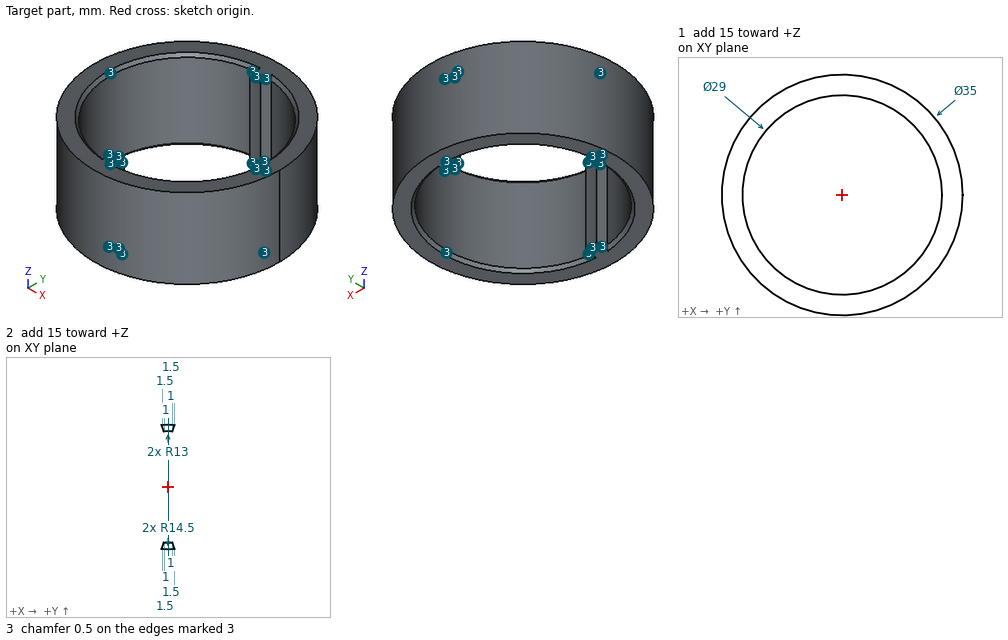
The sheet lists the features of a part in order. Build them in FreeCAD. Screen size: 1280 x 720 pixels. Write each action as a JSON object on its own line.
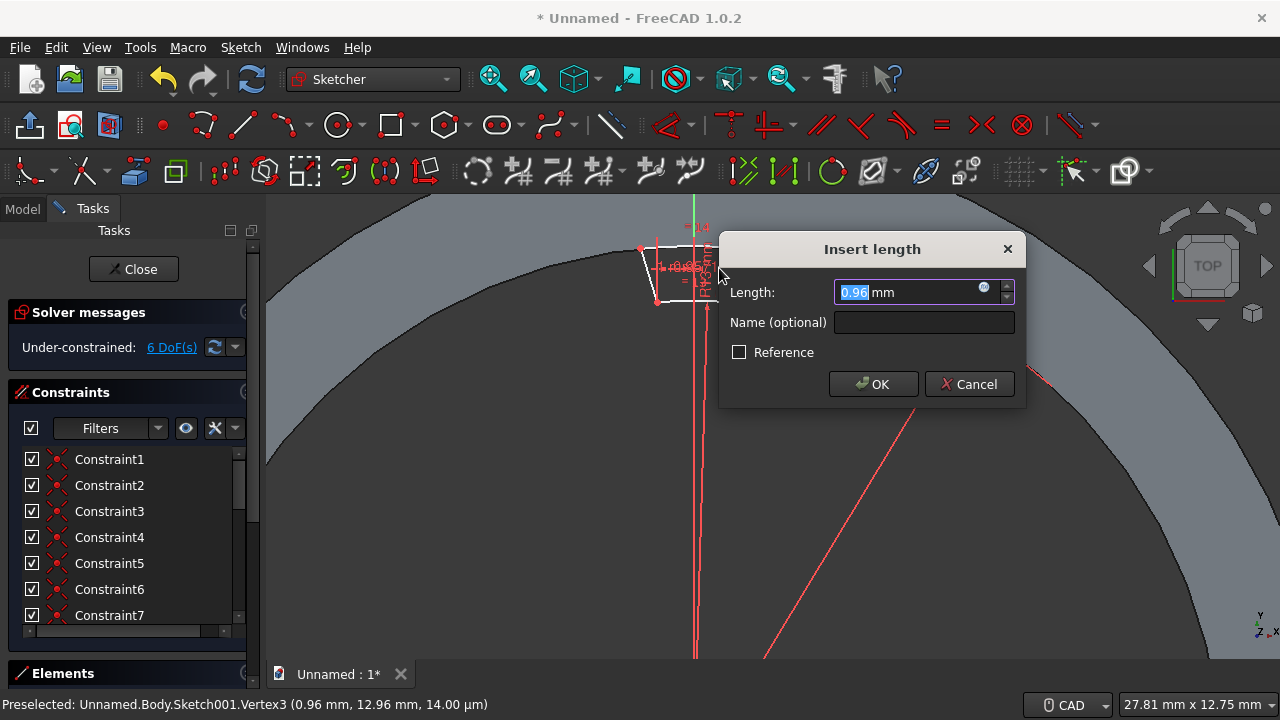
{"action": "type", "text": "1"}
{"action": "key", "text": "Return"}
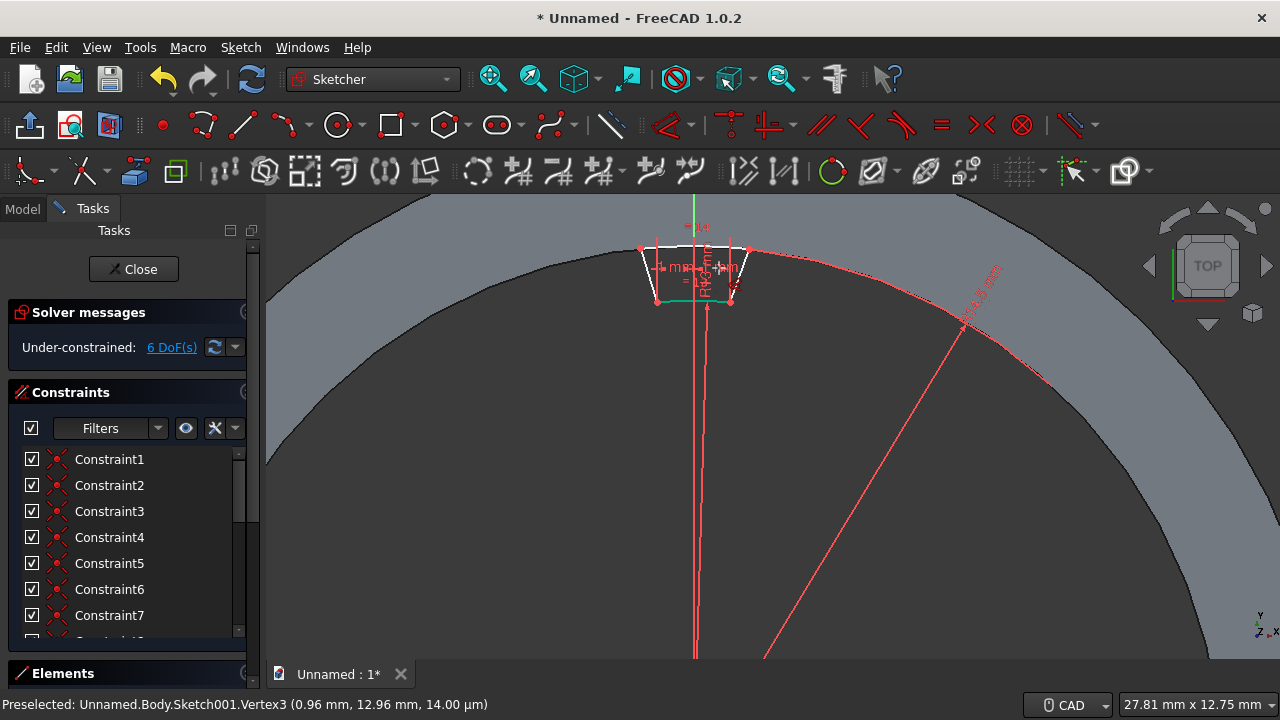
{"action": "scroll", "coordinate": [709, 276], "scroll_direction": "down", "scroll_amount": 6}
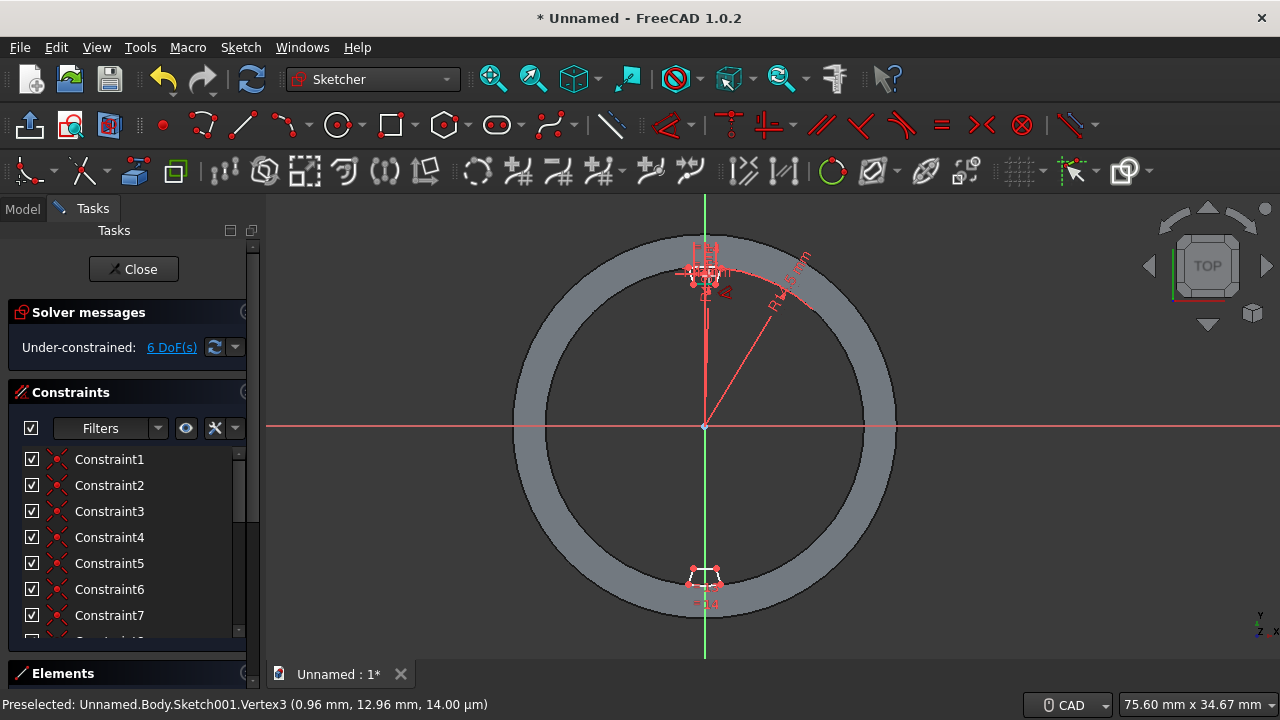
{"action": "scroll", "coordinate": [716, 569], "scroll_direction": "up", "scroll_amount": 7}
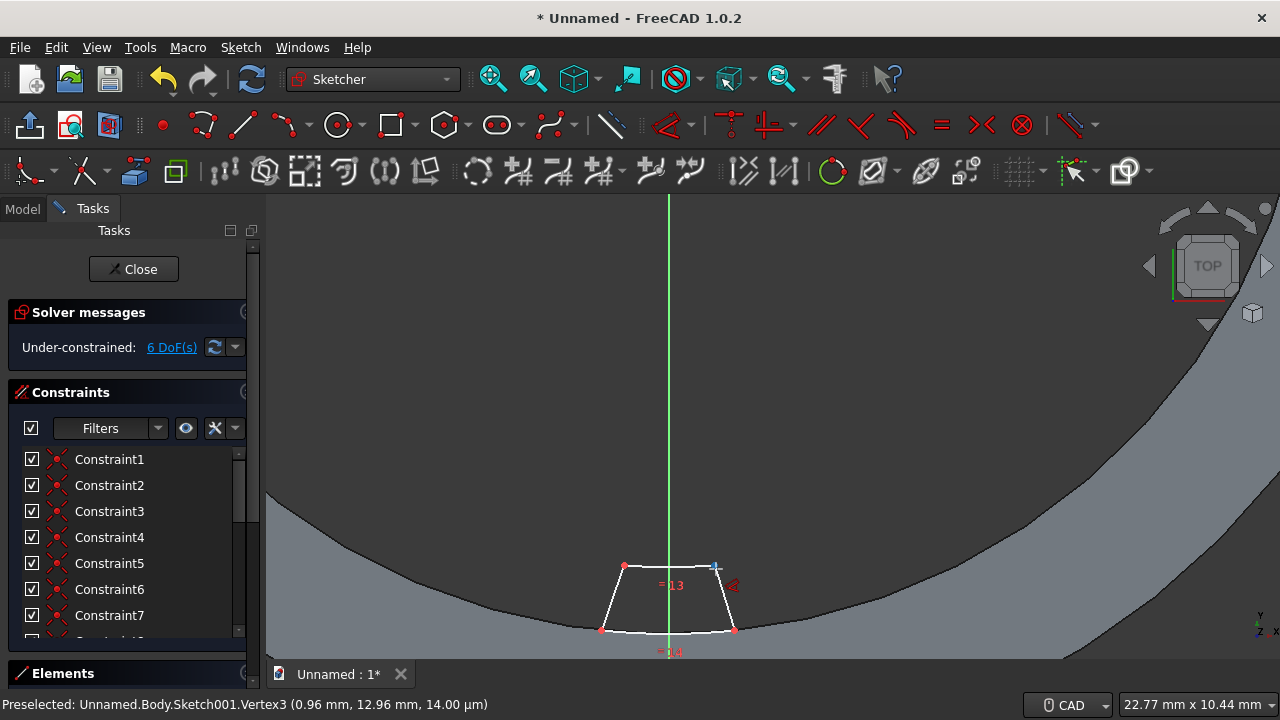
{"action": "left_click", "coordinate": [715, 565]}
{"action": "left_click", "coordinate": [692, 599]}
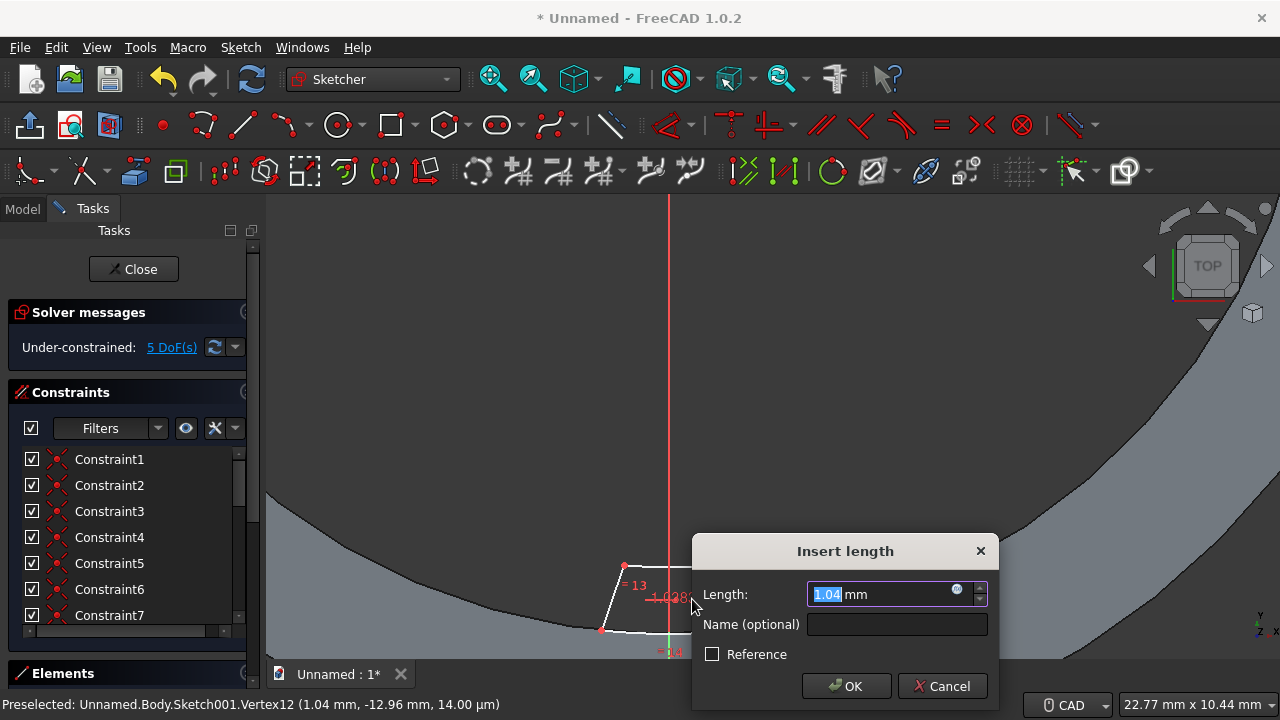
{"action": "type", "text": "1"}
{"action": "key", "text": "Return"}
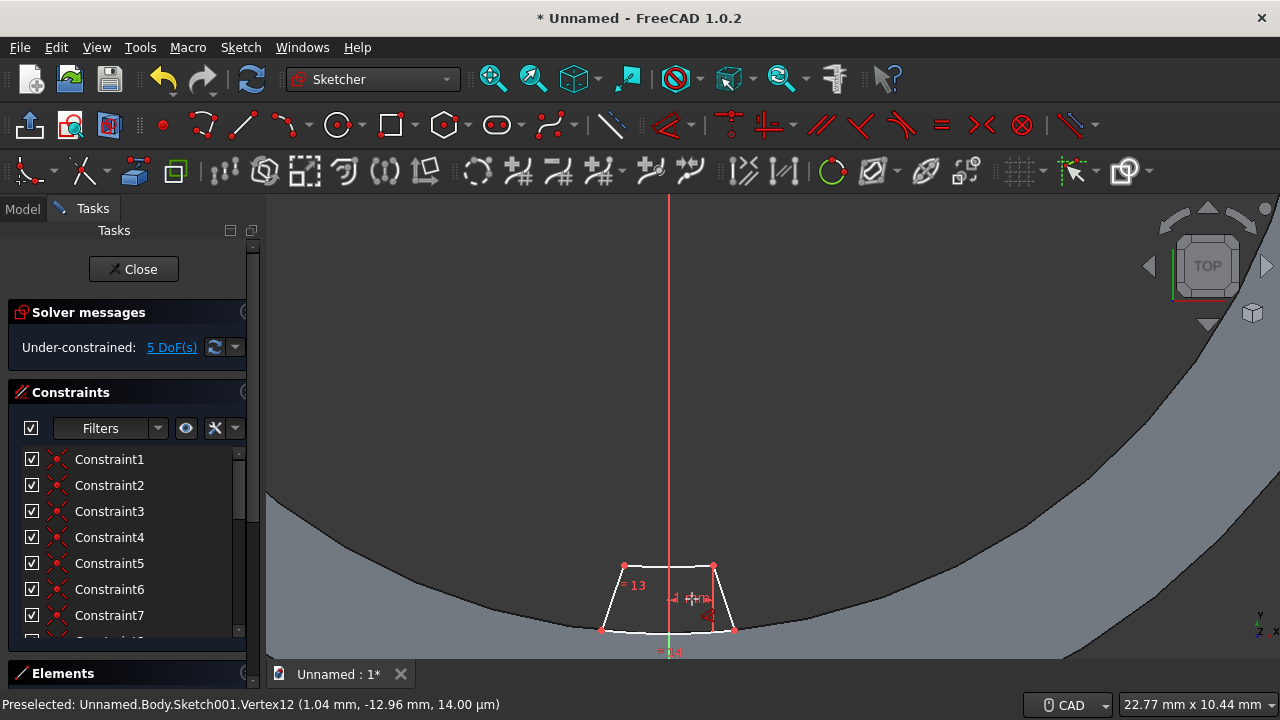
{"action": "left_click", "coordinate": [624, 565]}
{"action": "left_click", "coordinate": [646, 599]}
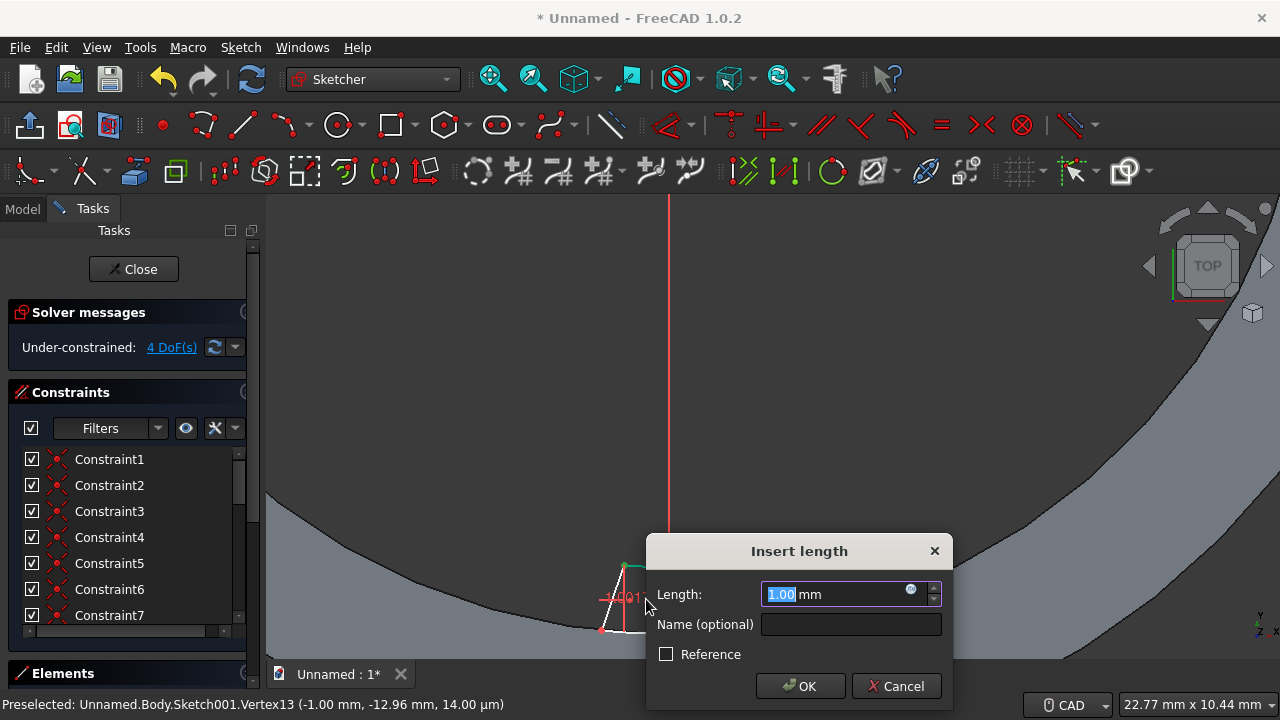
{"action": "type", "text": "1"}
{"action": "key", "text": "Return"}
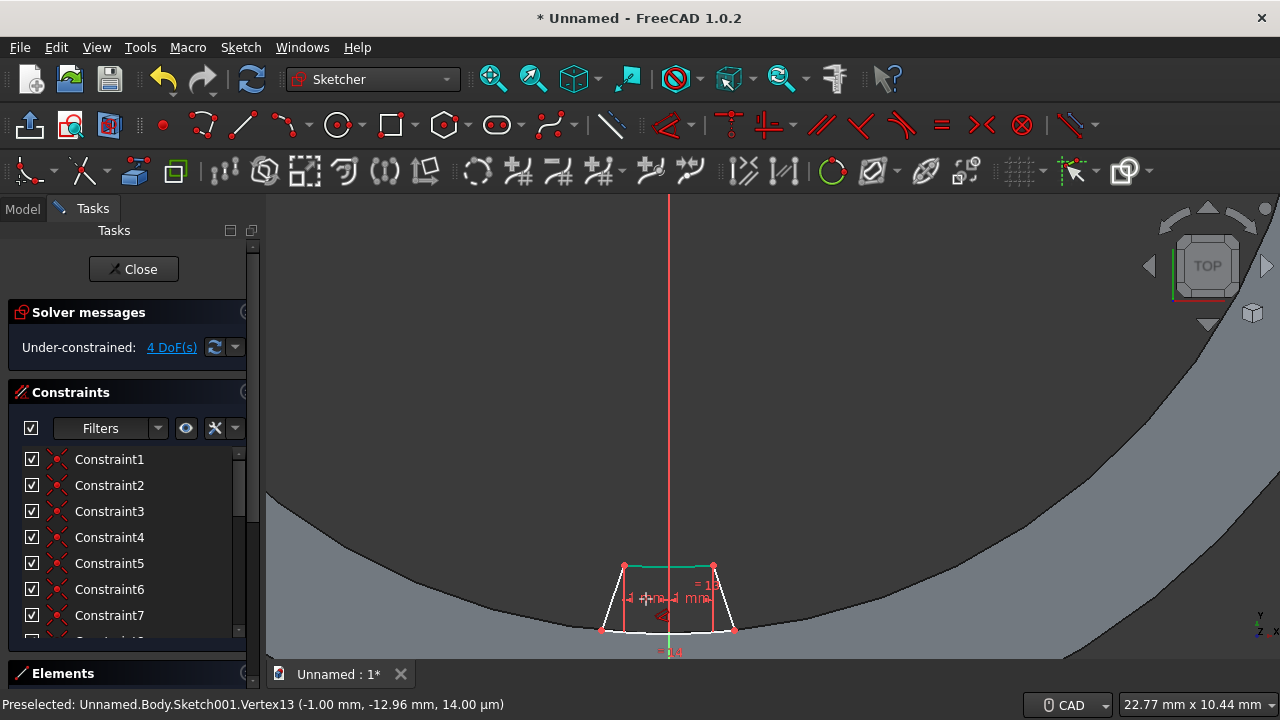
{"action": "scroll", "coordinate": [716, 570], "scroll_direction": "down", "scroll_amount": 7}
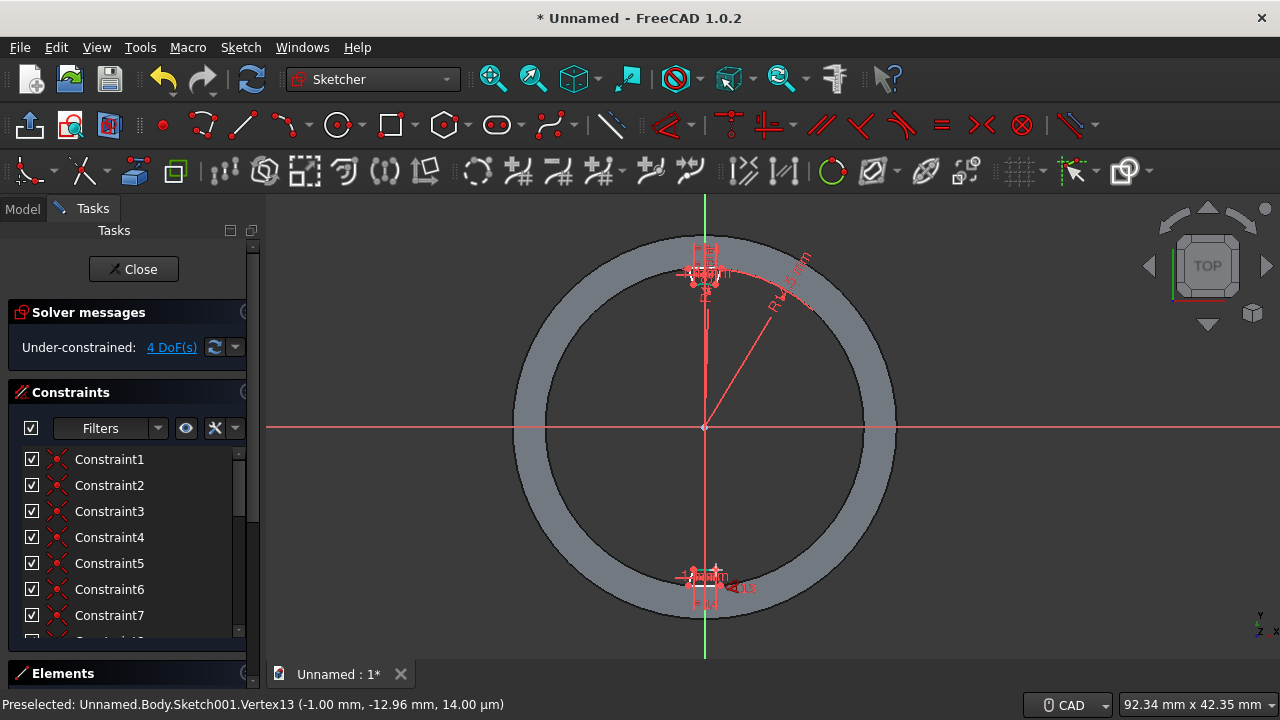
{"action": "scroll", "coordinate": [689, 269], "scroll_direction": "up", "scroll_amount": 5}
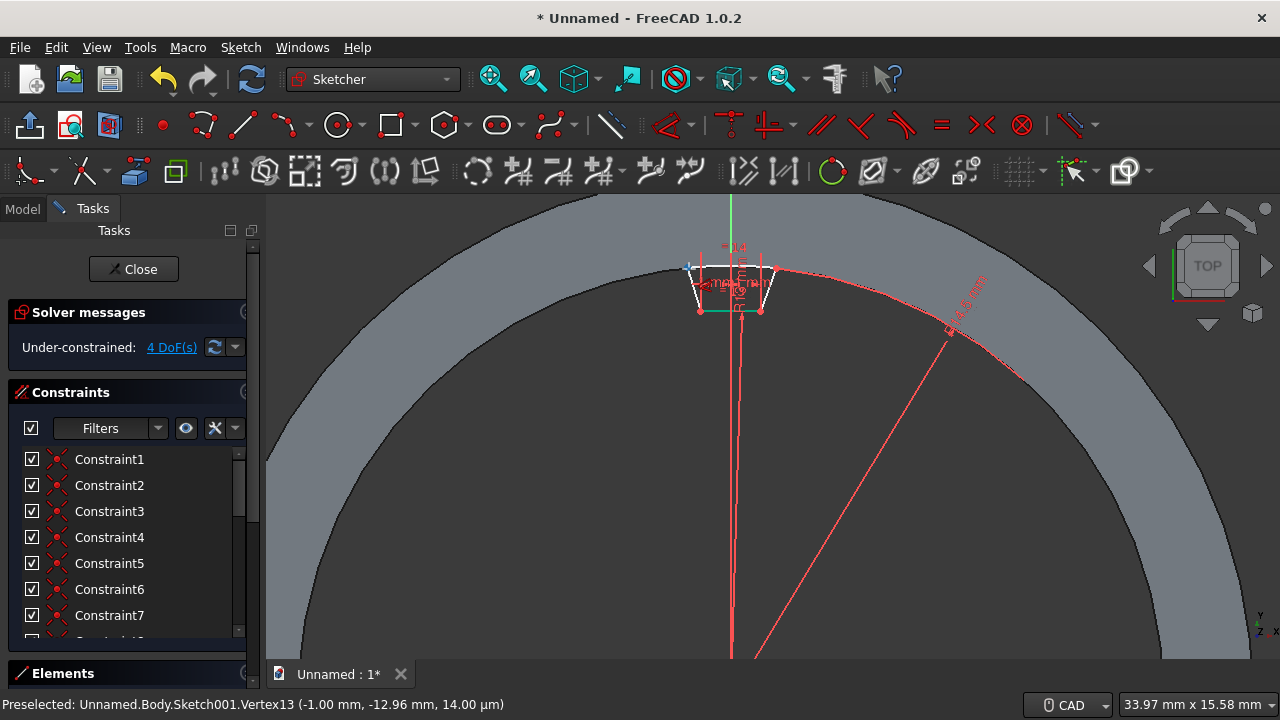
{"action": "left_click", "coordinate": [688, 268]}
{"action": "left_click", "coordinate": [709, 234]}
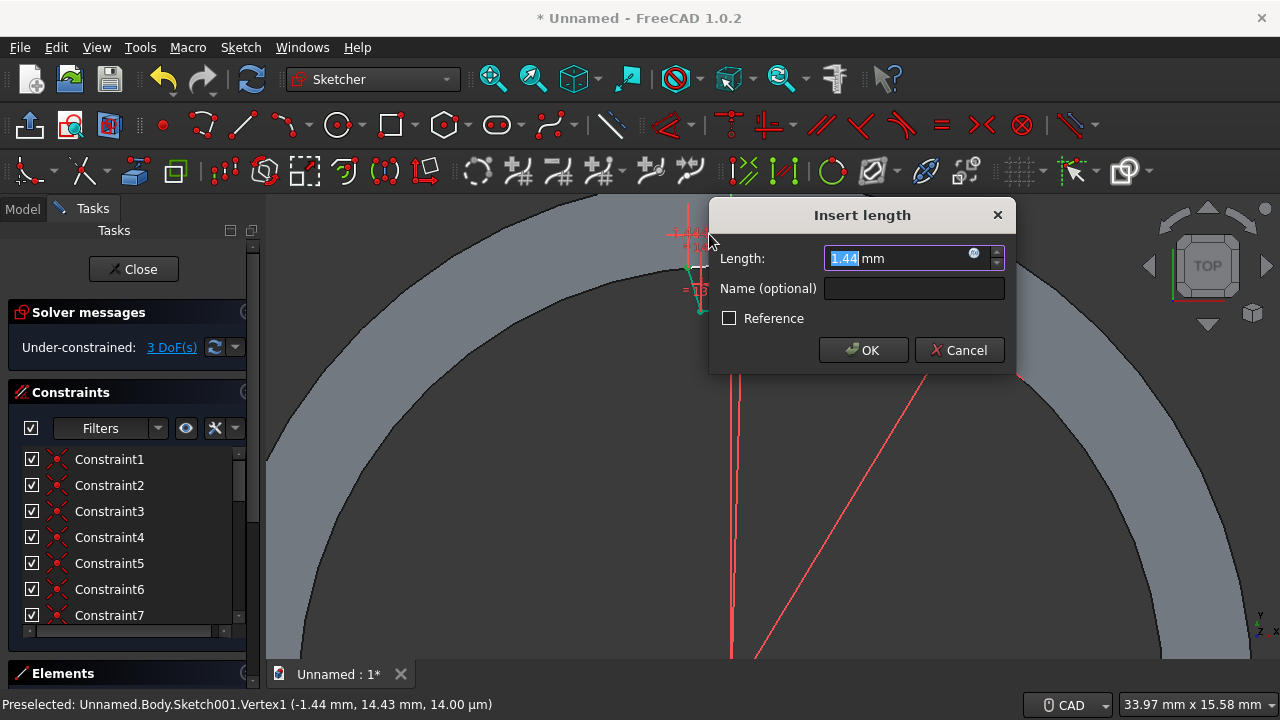
{"action": "type", "text": "1.5"}
{"action": "key", "text": "Return"}